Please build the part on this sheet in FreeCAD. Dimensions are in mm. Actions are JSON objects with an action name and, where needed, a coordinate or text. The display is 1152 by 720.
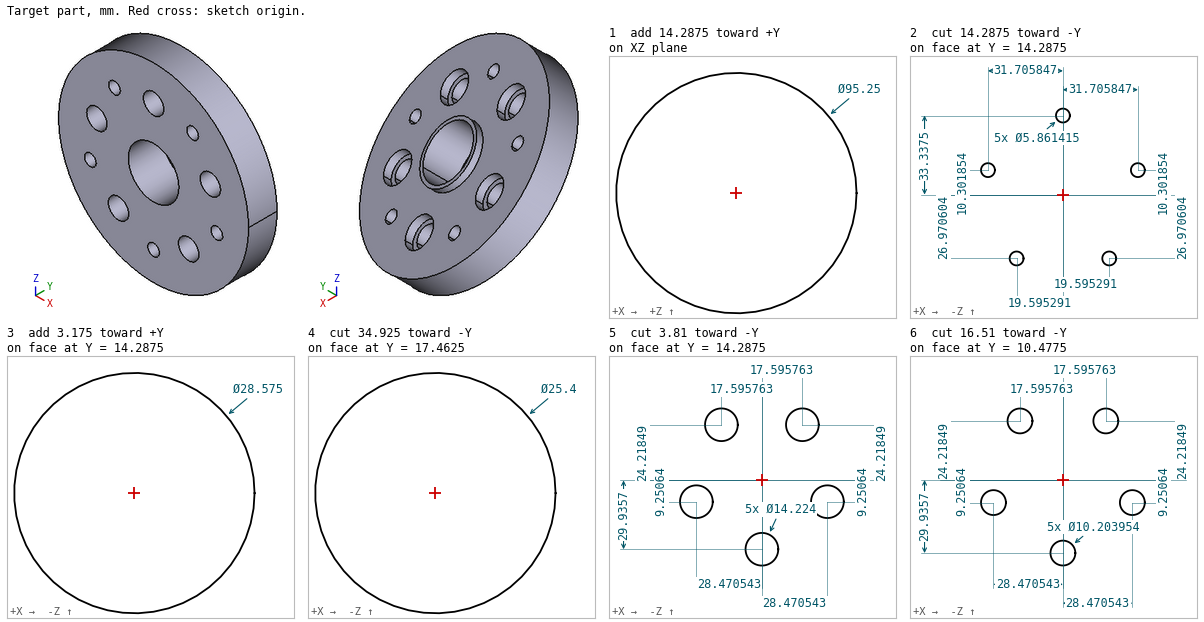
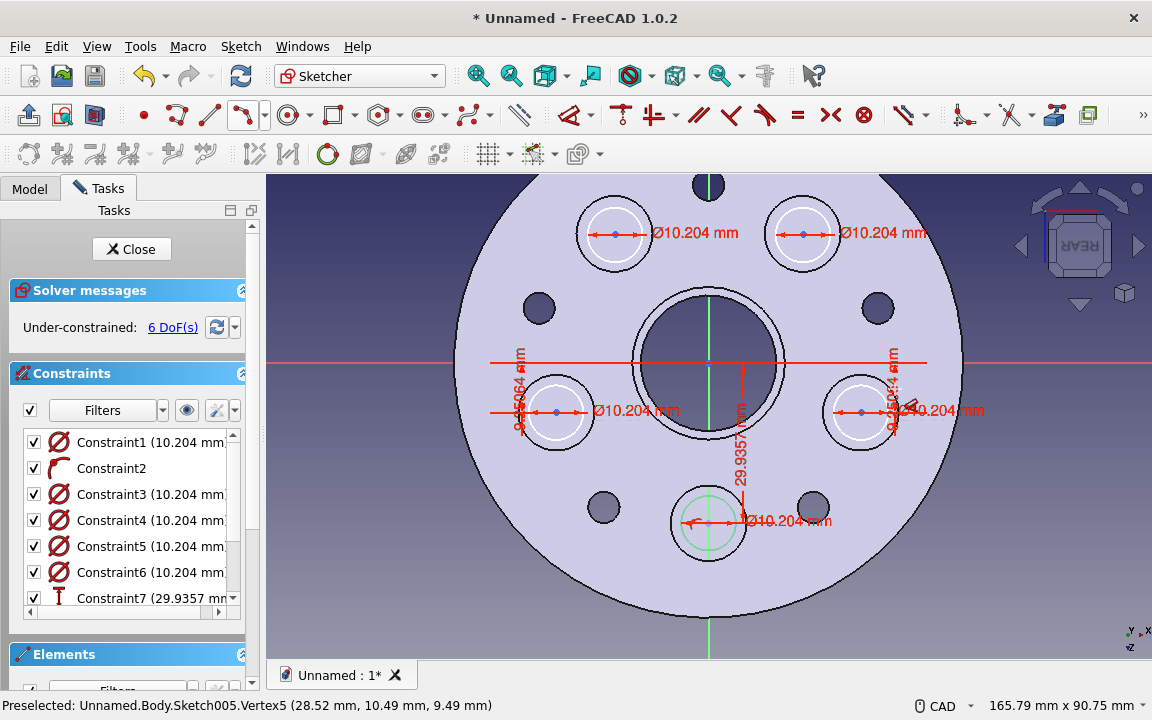
{"action": "left_click", "coordinate": [615, 235]}
{"action": "left_click", "coordinate": [581, 299]}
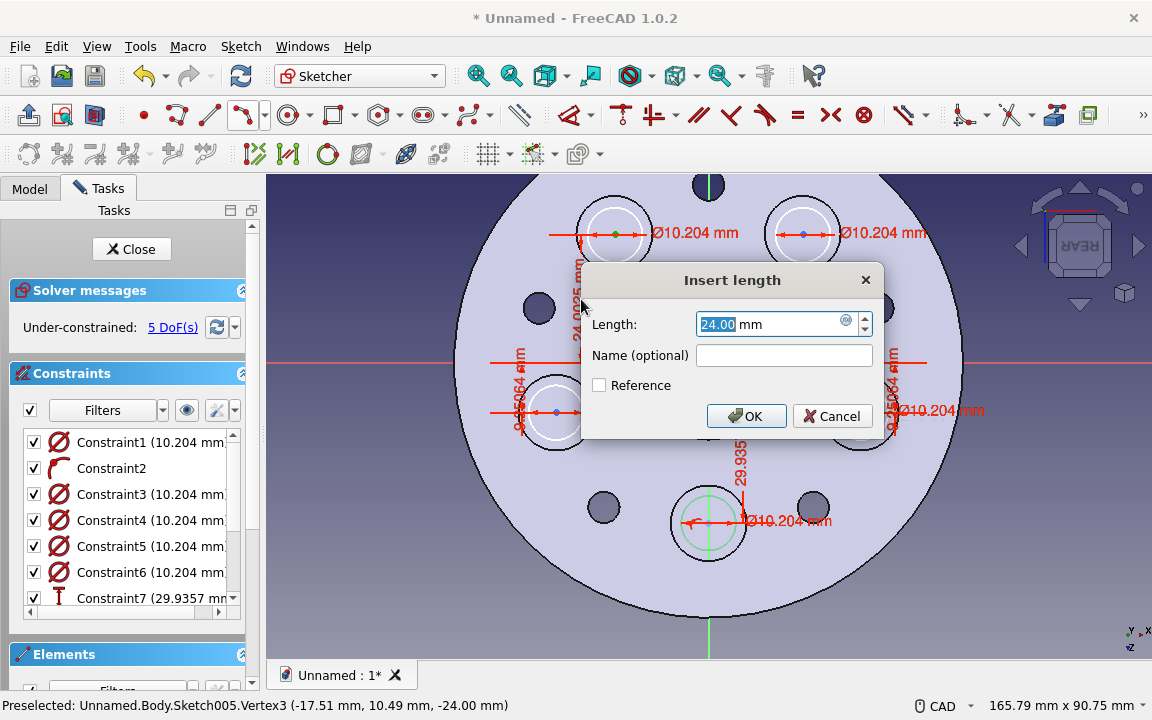
{"action": "type", "text": "24.21849"}
{"action": "key", "text": "Return"}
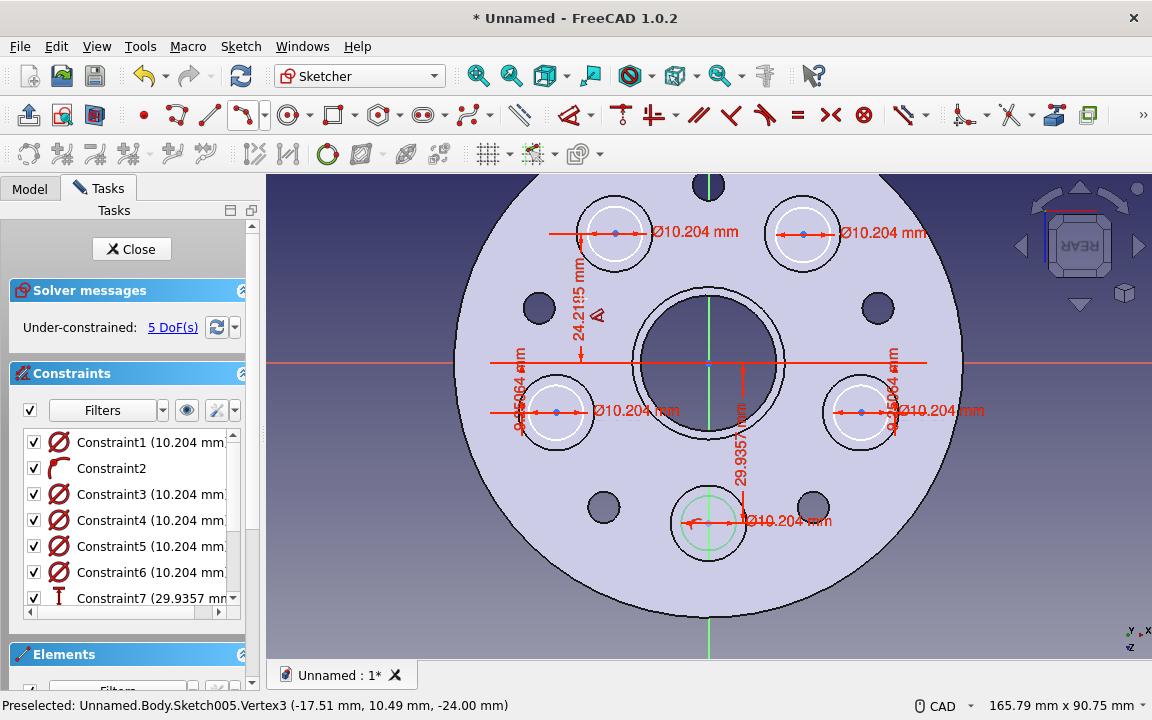
{"action": "left_click", "coordinate": [803, 235]}
{"action": "left_click", "coordinate": [837, 299]}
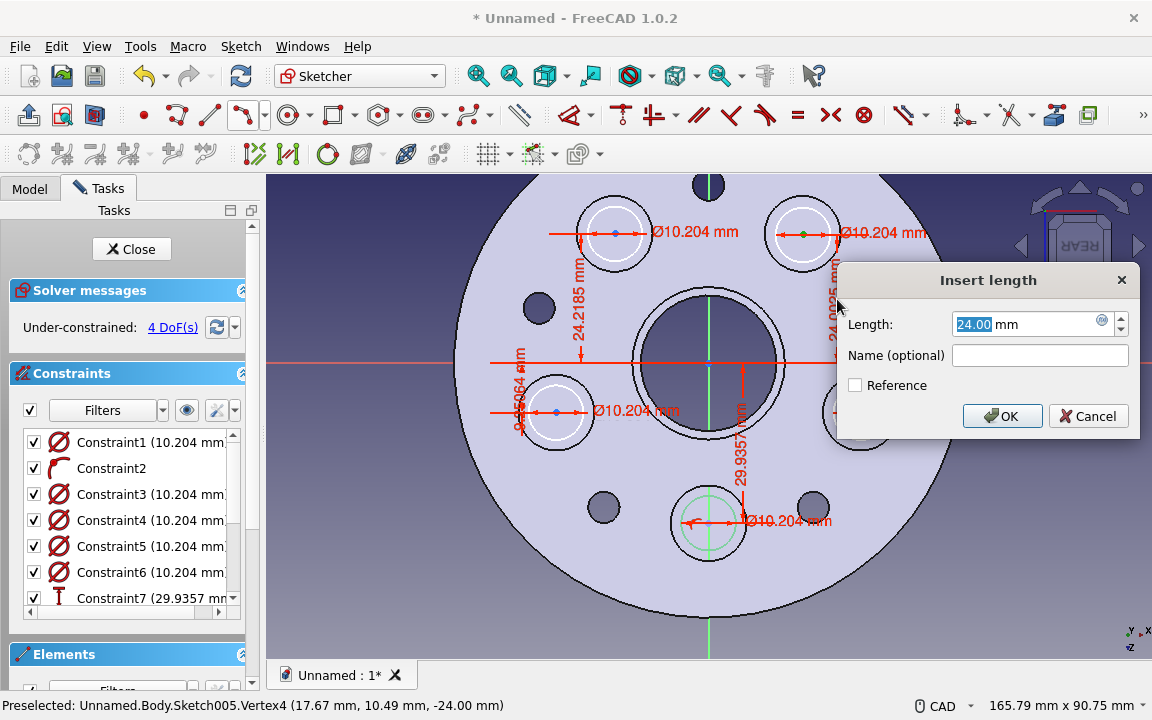
{"action": "type", "text": "24.21849"}
{"action": "key", "text": "Return"}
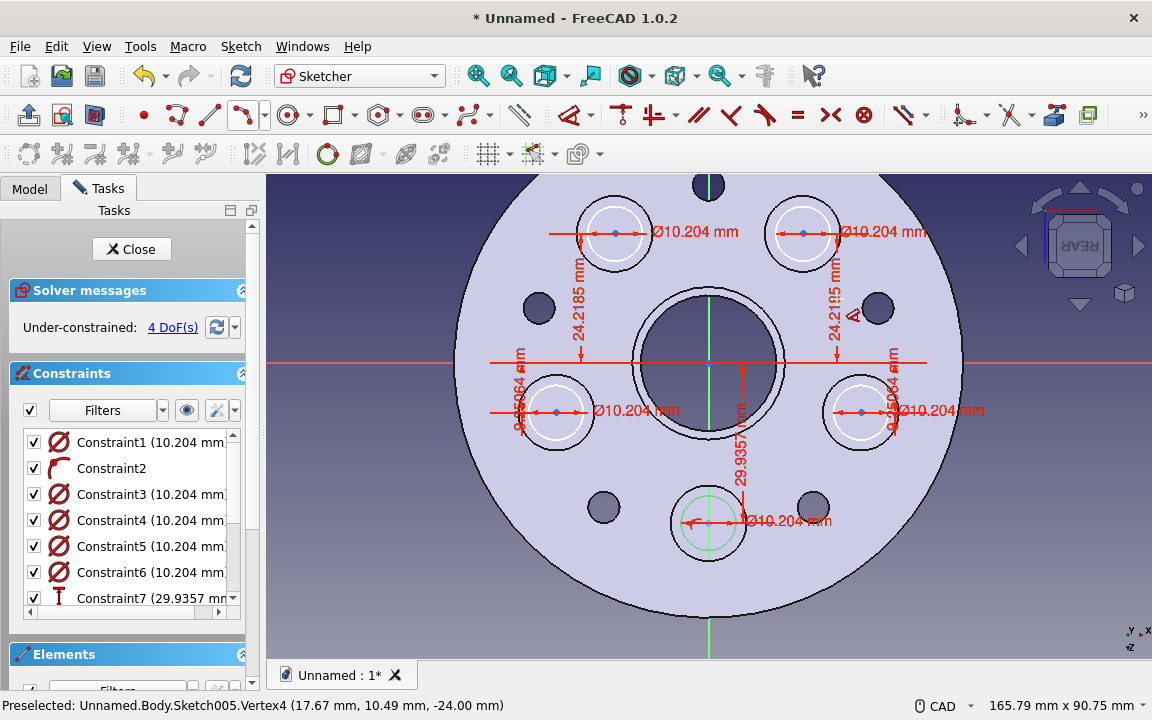
{"action": "left_click", "coordinate": [556, 413]}
{"action": "left_click", "coordinate": [632, 447]}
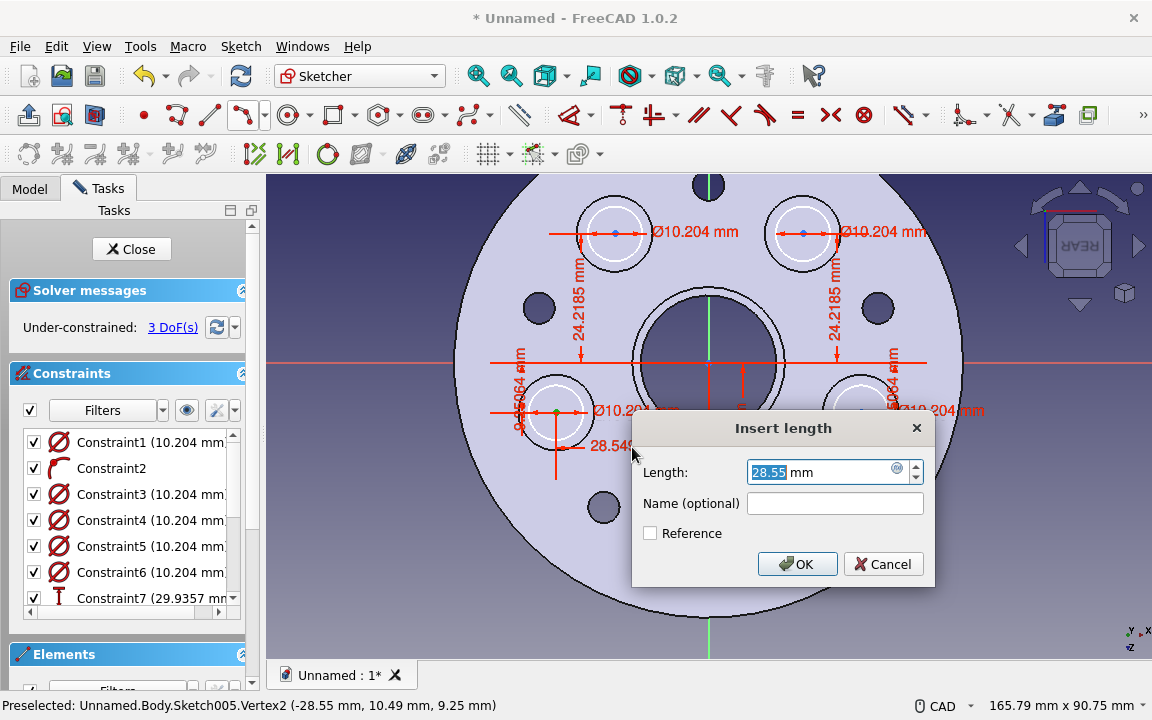
{"action": "type", "text": "28.470543"}
{"action": "key", "text": "Return"}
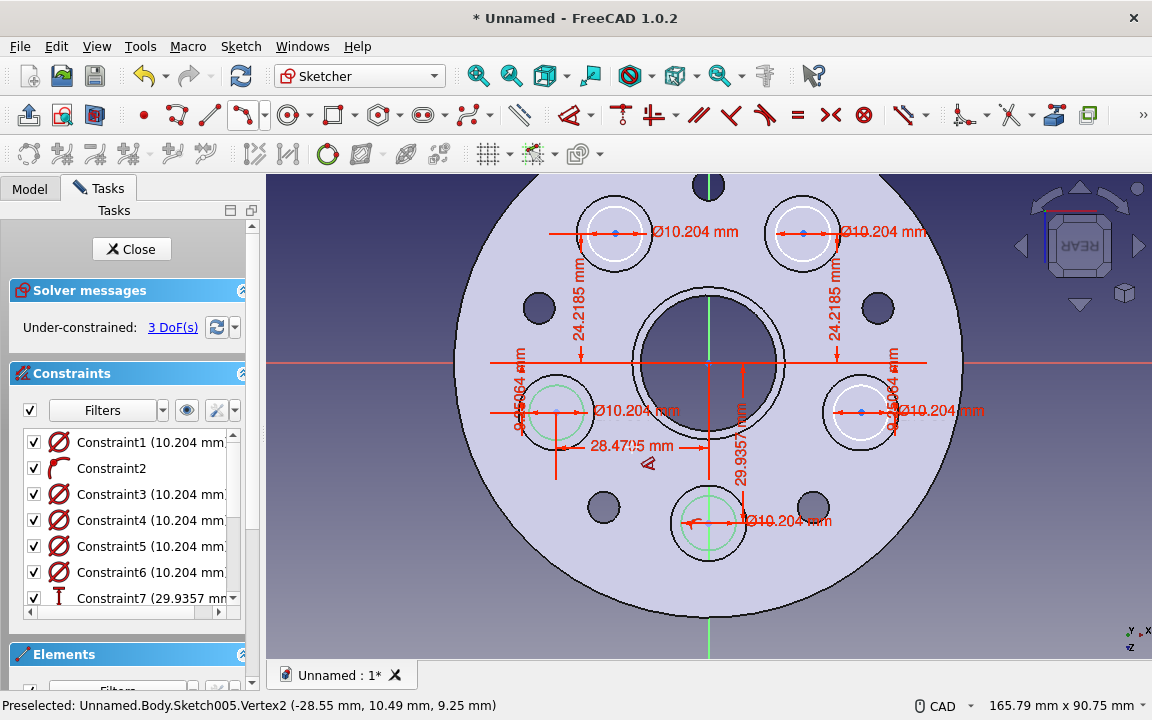
{"action": "left_click", "coordinate": [615, 234]}
{"action": "left_click", "coordinate": [662, 397]}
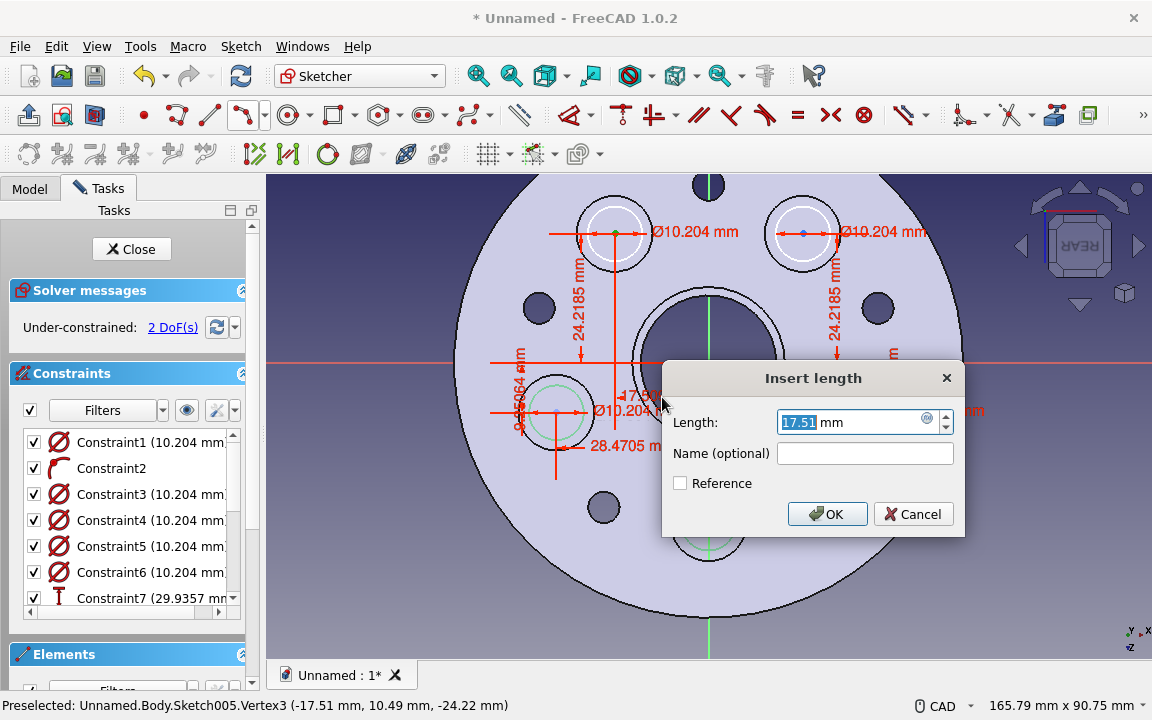
{"action": "type", "text": "17.595763"}
{"action": "key", "text": "Return"}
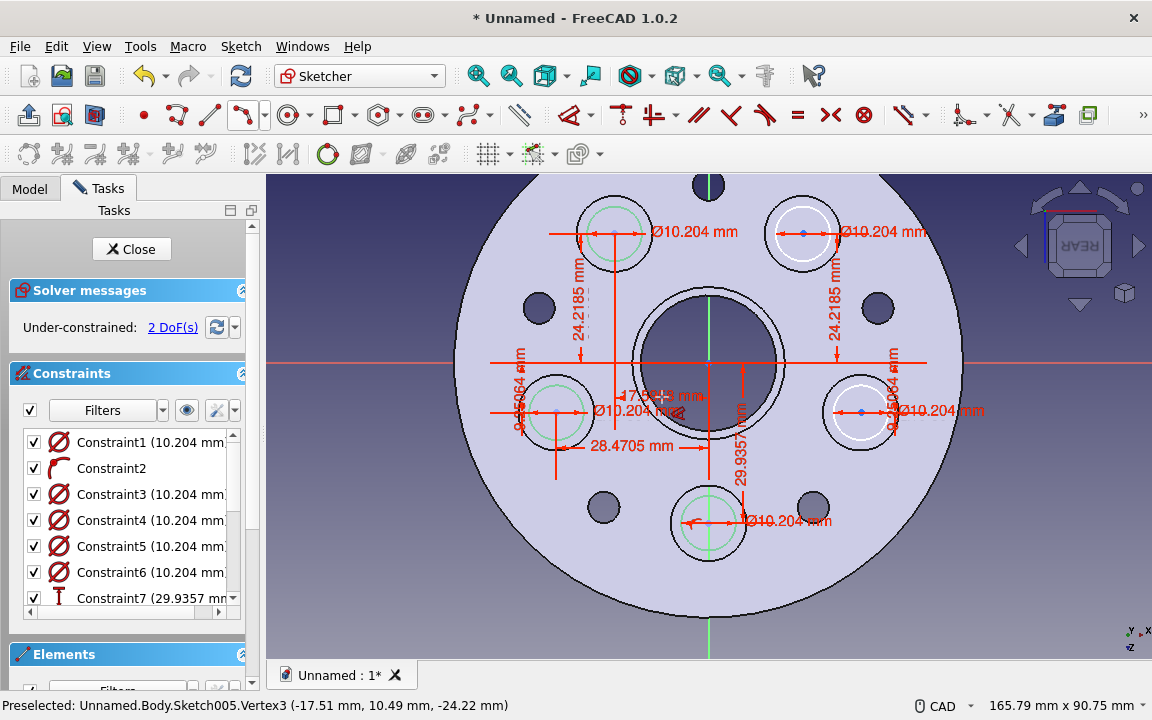
{"action": "left_click", "coordinate": [803, 234]}
{"action": "left_click", "coordinate": [756, 397]}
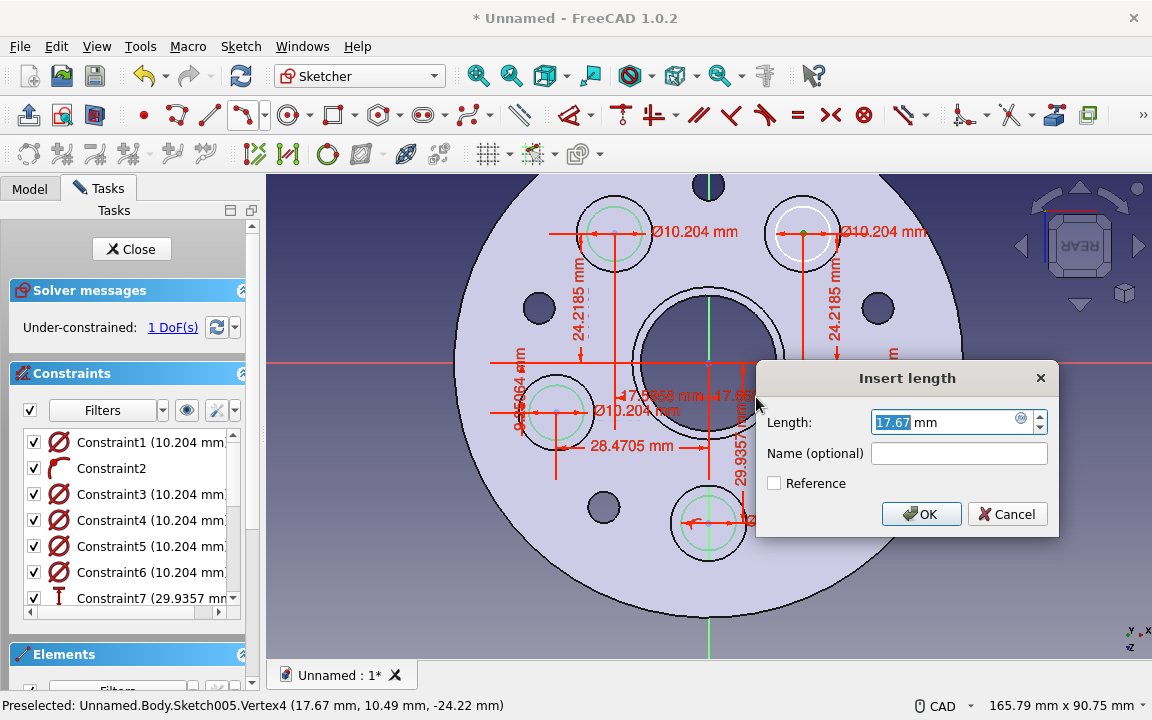
{"action": "type", "text": "17.595763"}
{"action": "key", "text": "Return"}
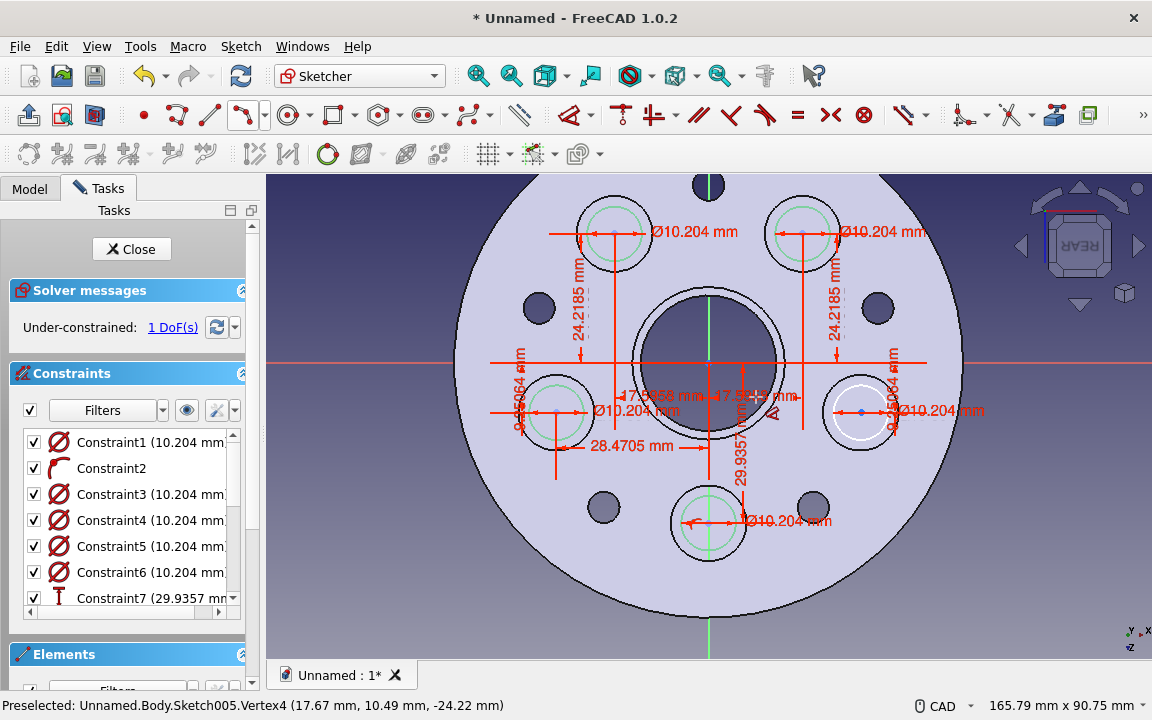
{"action": "left_click", "coordinate": [861, 413]}
{"action": "left_click", "coordinate": [820, 447]}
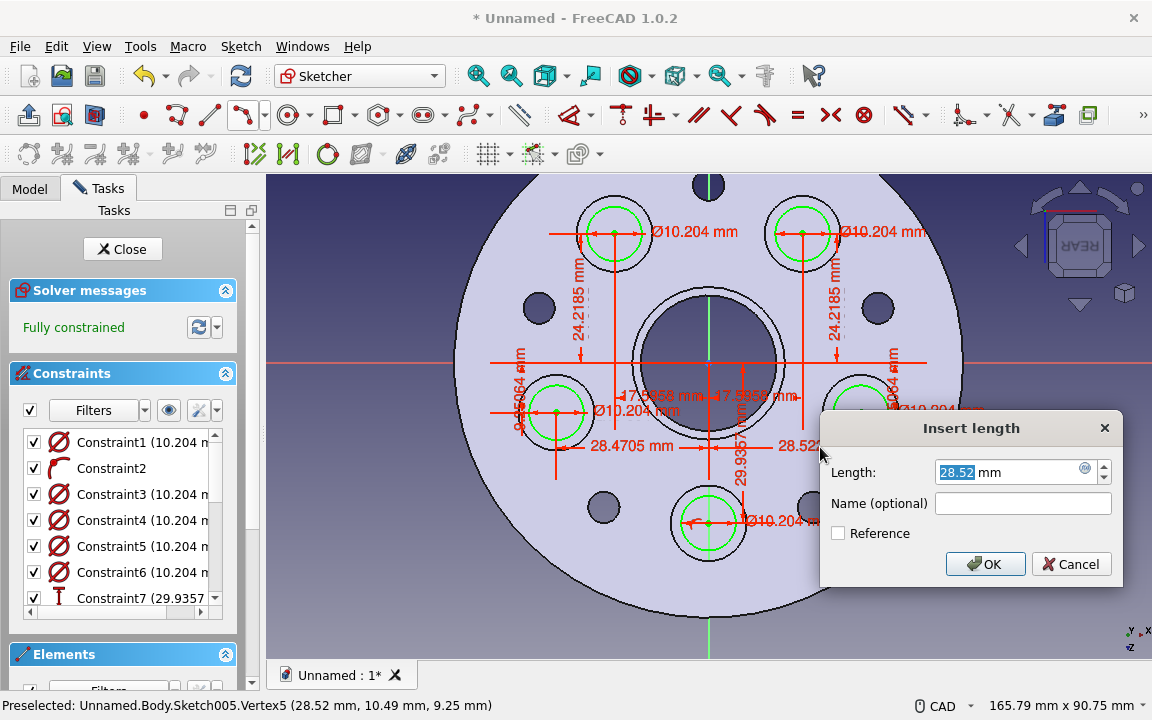
{"action": "type", "text": "28.470543"}
{"action": "key", "text": "Return"}
{"action": "key", "text": "Escape"}